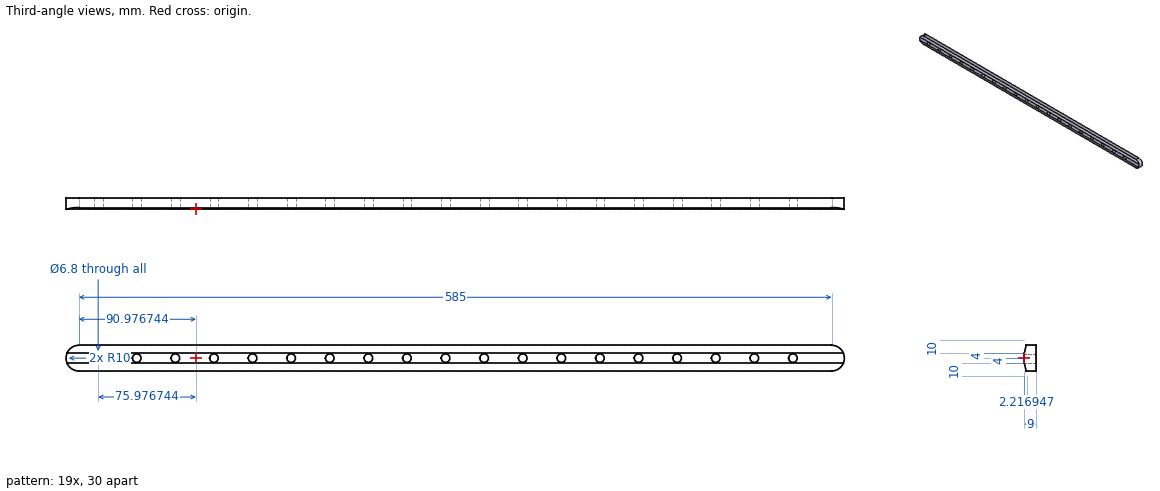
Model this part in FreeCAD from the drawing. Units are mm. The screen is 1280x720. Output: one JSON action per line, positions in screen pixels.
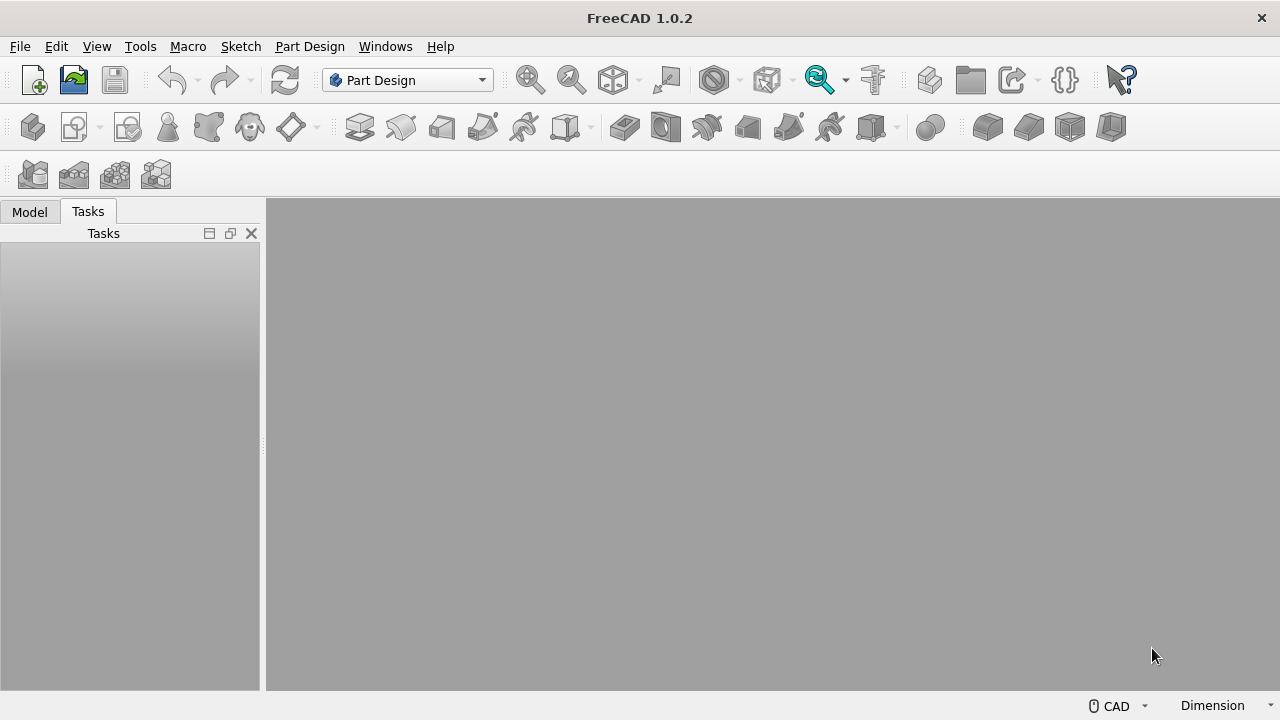
{"action": "left_click", "coordinate": [33, 80]}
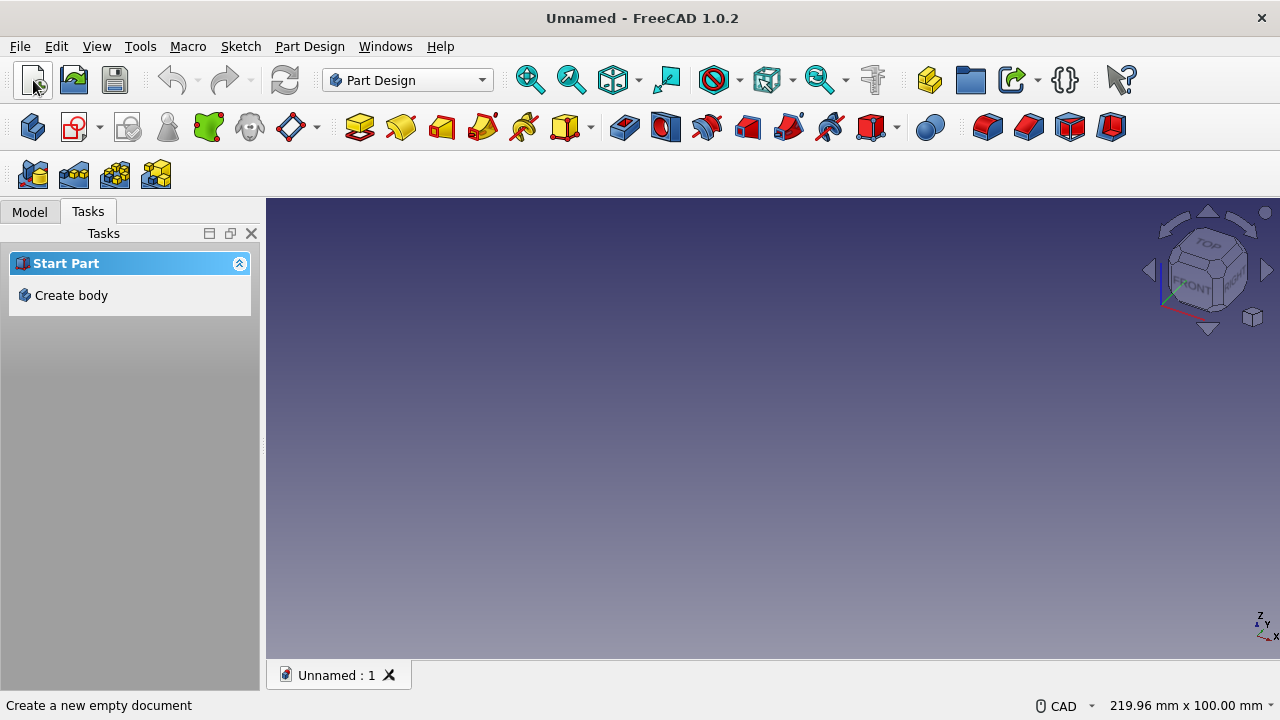
{"action": "left_click", "coordinate": [74, 128]}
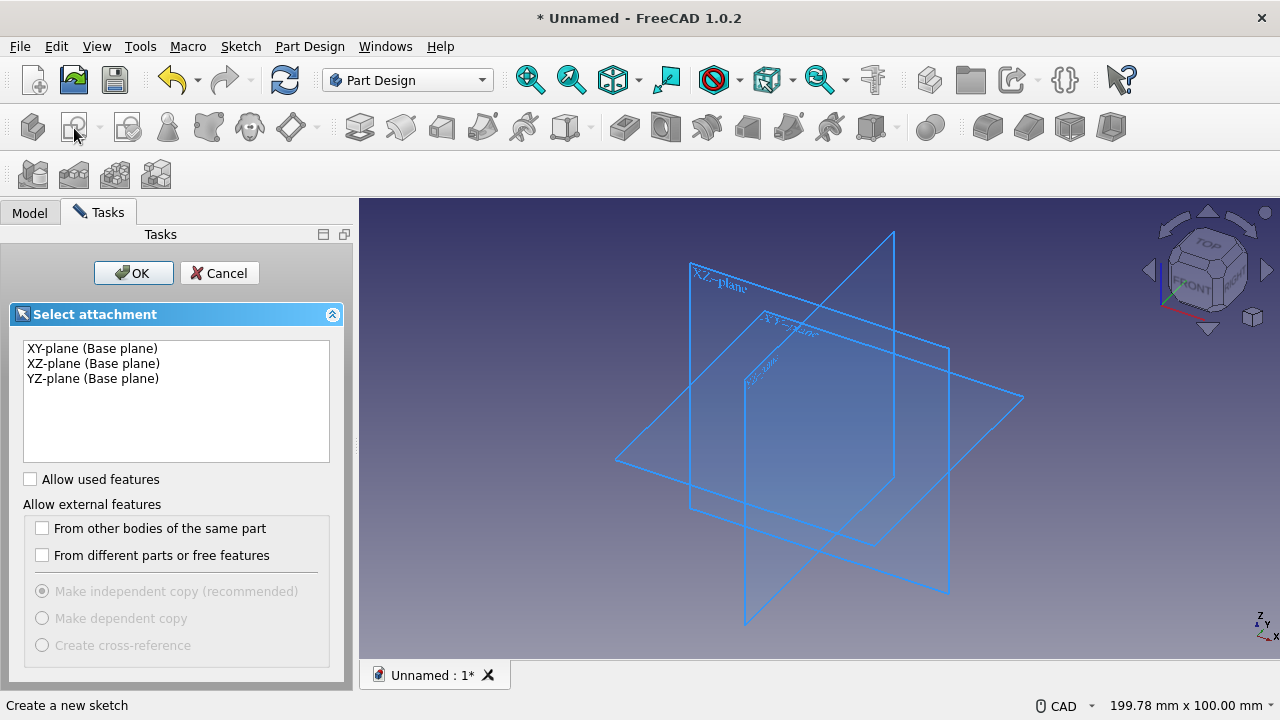
{"action": "left_click", "coordinate": [84, 364]}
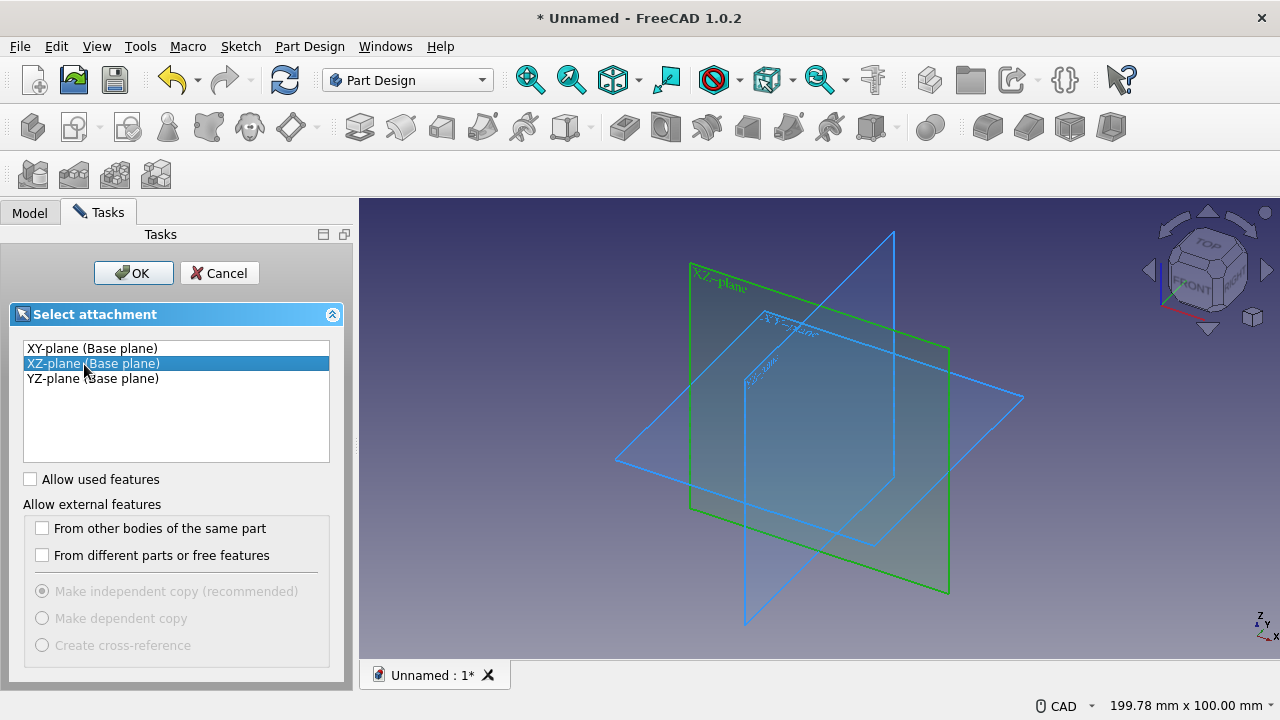
{"action": "left_click", "coordinate": [134, 273]}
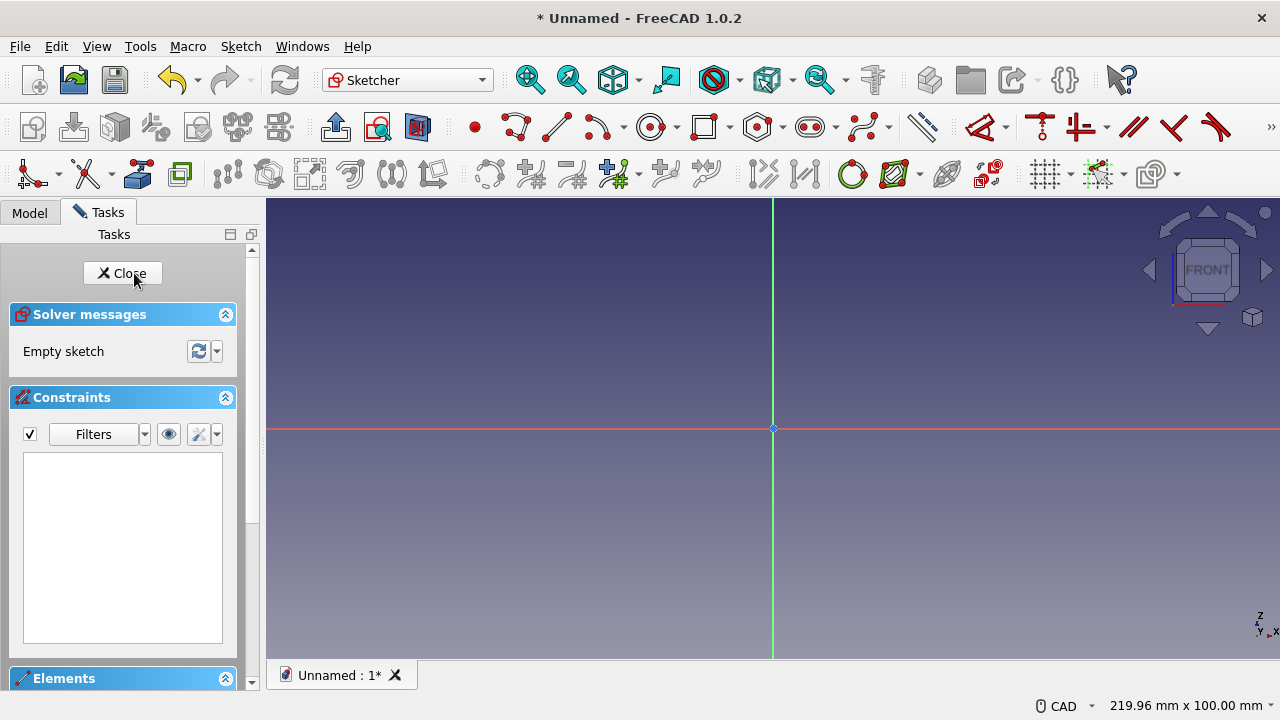
{"action": "scroll", "coordinate": [452, 428], "scroll_direction": "down", "scroll_amount": 8}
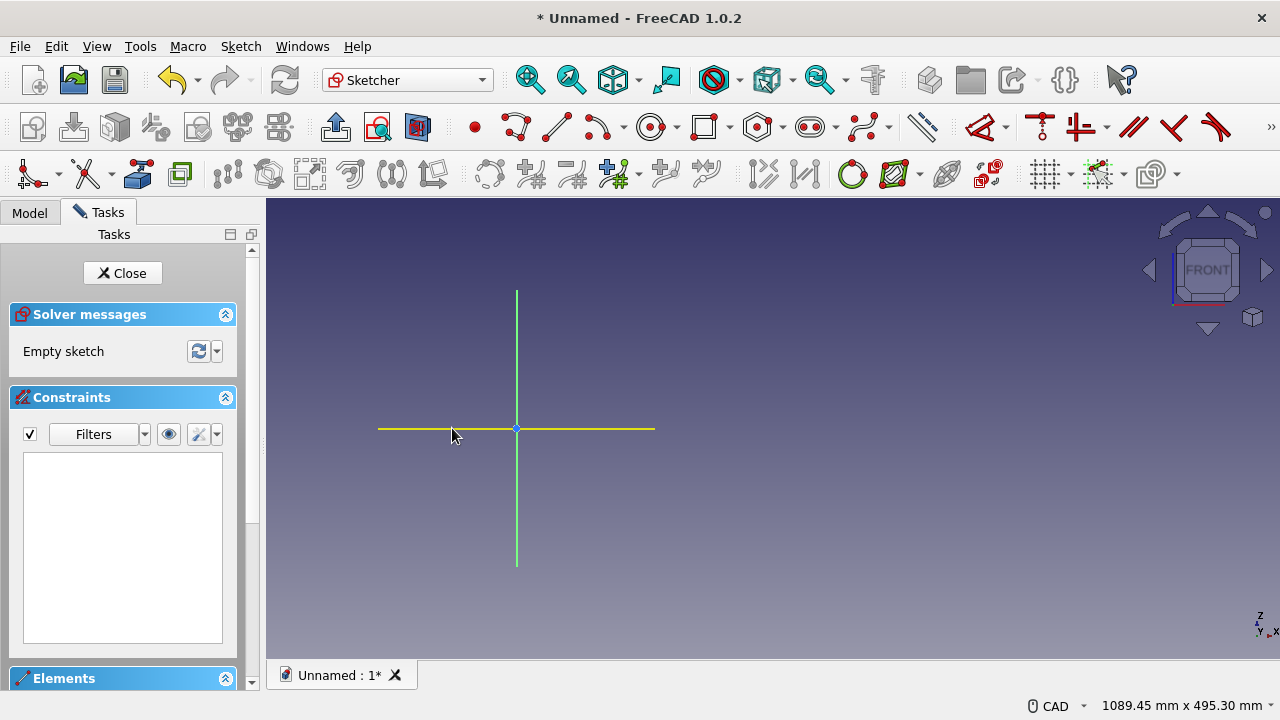
{"action": "left_click", "coordinate": [810, 128]}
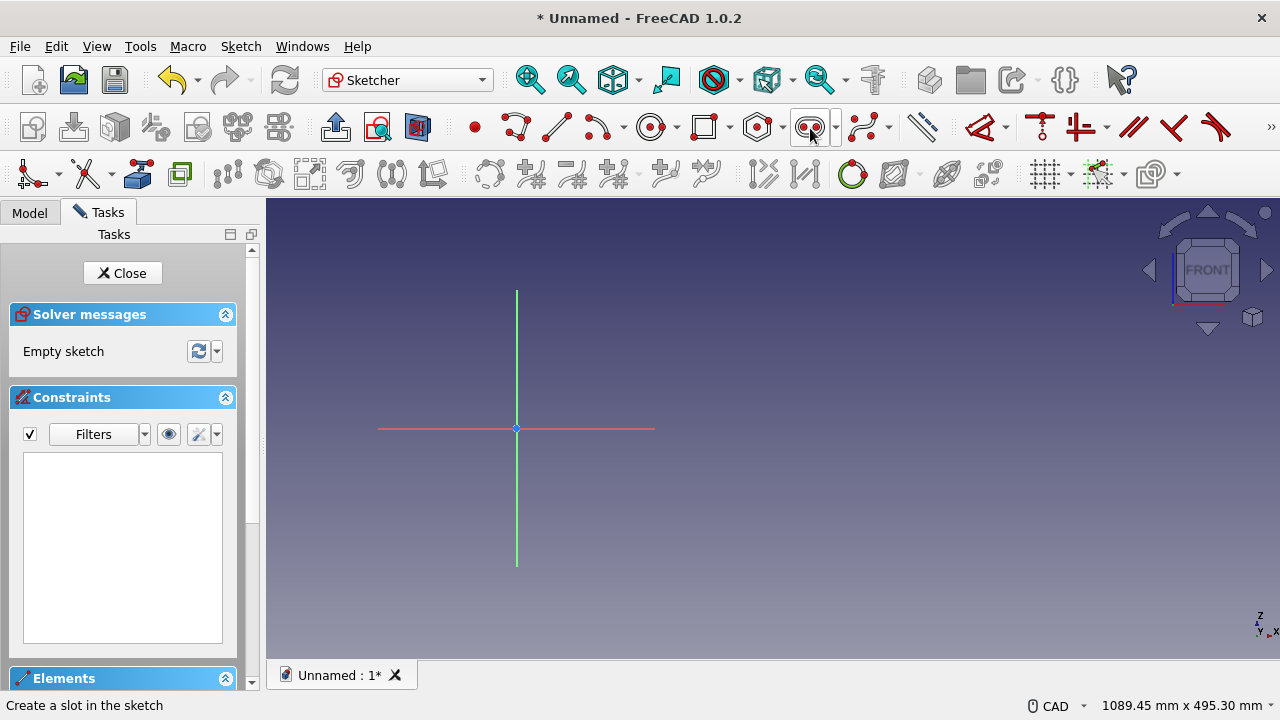
{"action": "scroll", "coordinate": [432, 428], "scroll_direction": "up", "scroll_amount": 5}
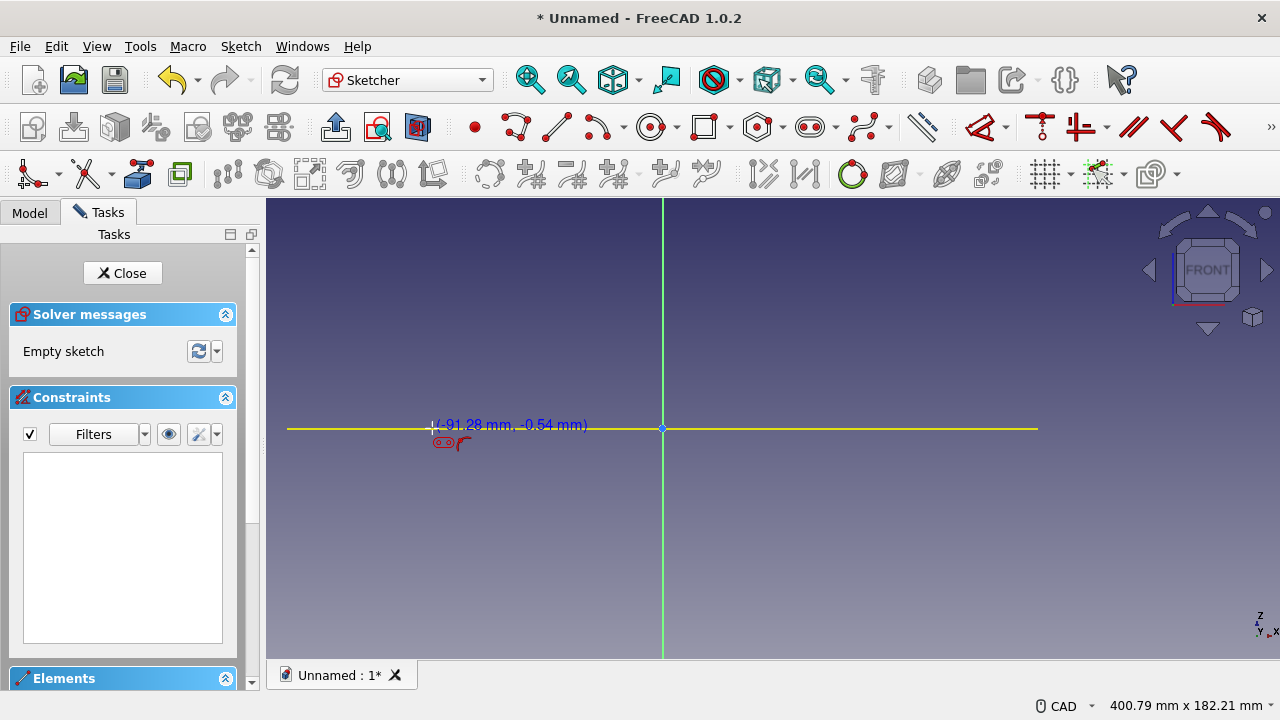
{"action": "left_click", "coordinate": [432, 428]}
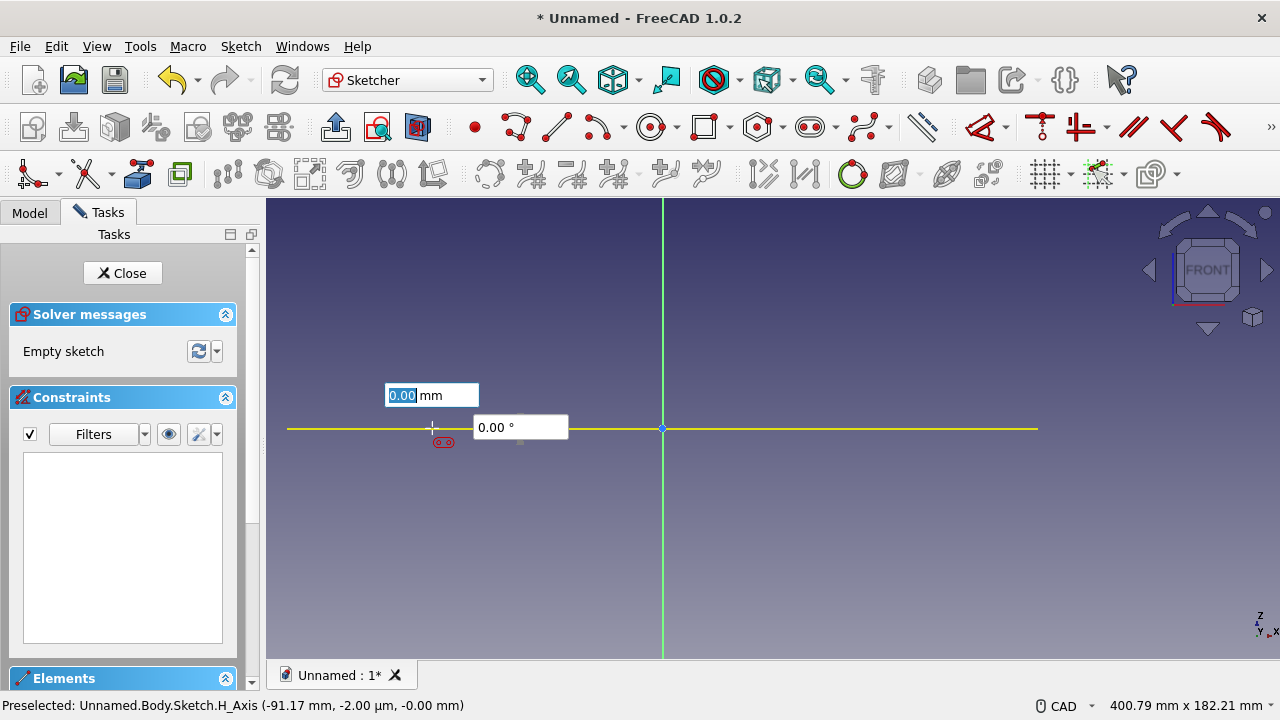
{"action": "scroll", "coordinate": [432, 428], "scroll_direction": "down", "scroll_amount": 5}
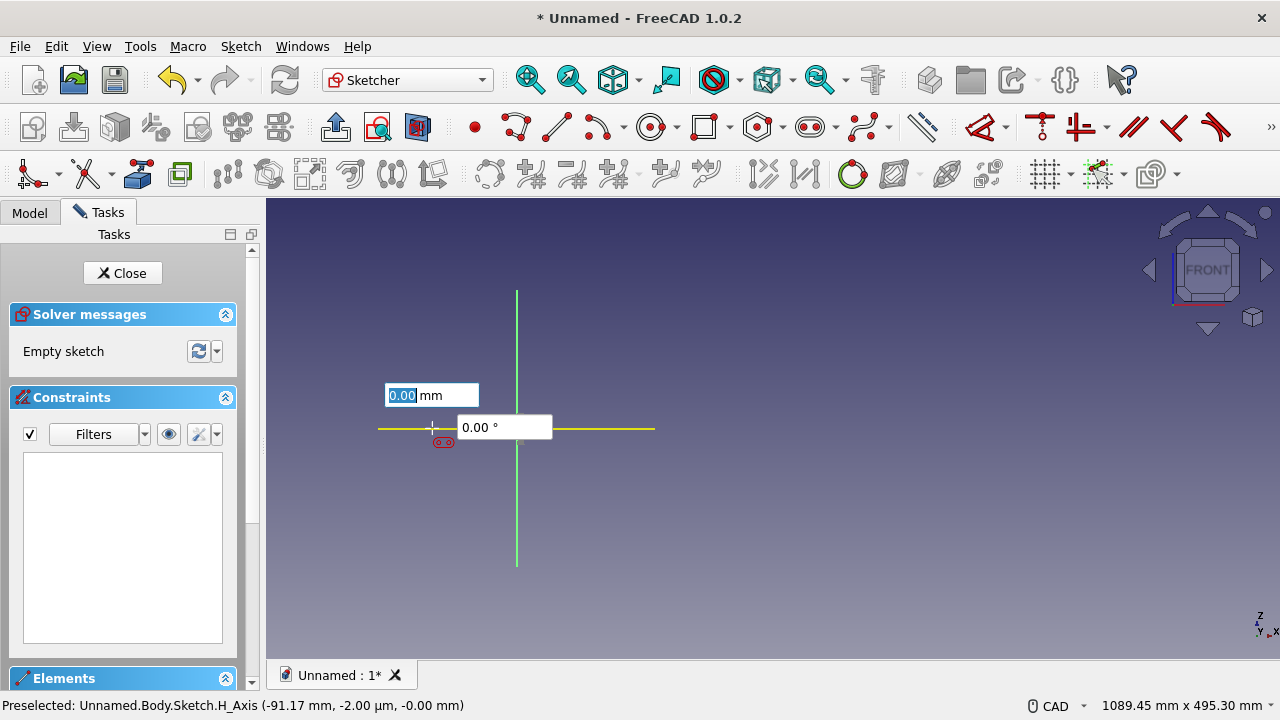
{"action": "left_click", "coordinate": [977, 420]}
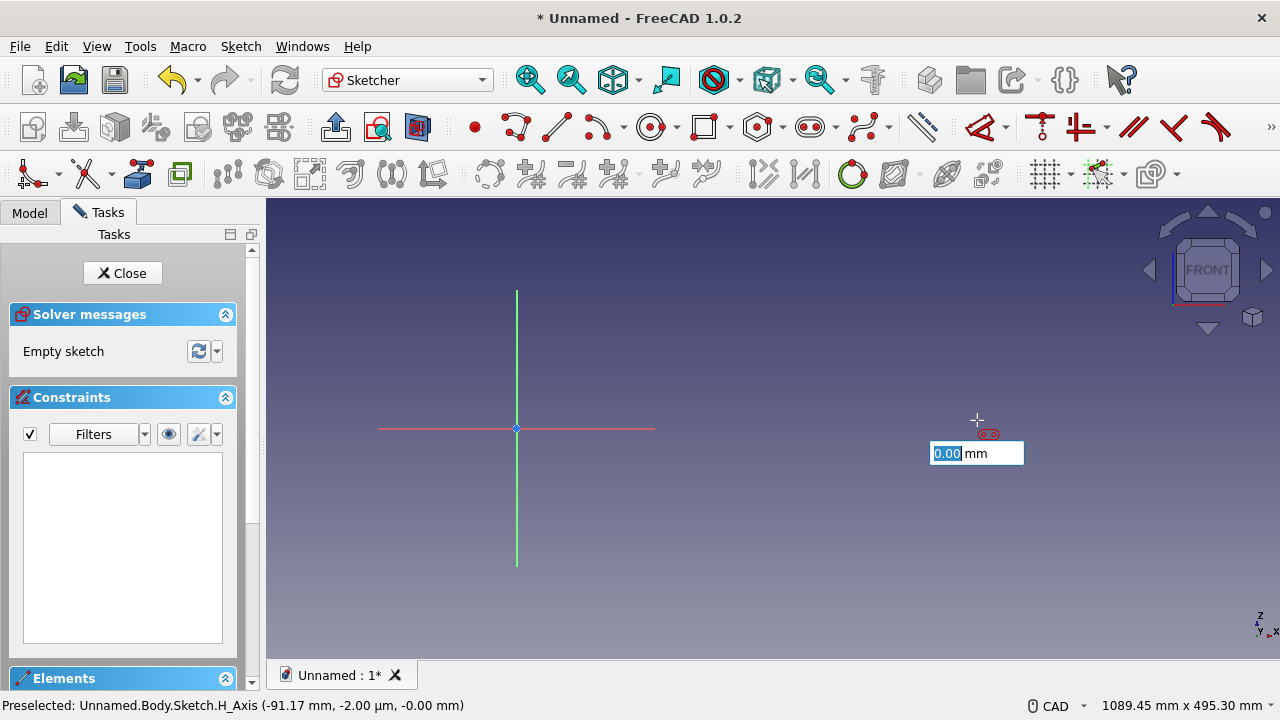
{"action": "scroll", "coordinate": [705, 438], "scroll_direction": "up", "scroll_amount": 3}